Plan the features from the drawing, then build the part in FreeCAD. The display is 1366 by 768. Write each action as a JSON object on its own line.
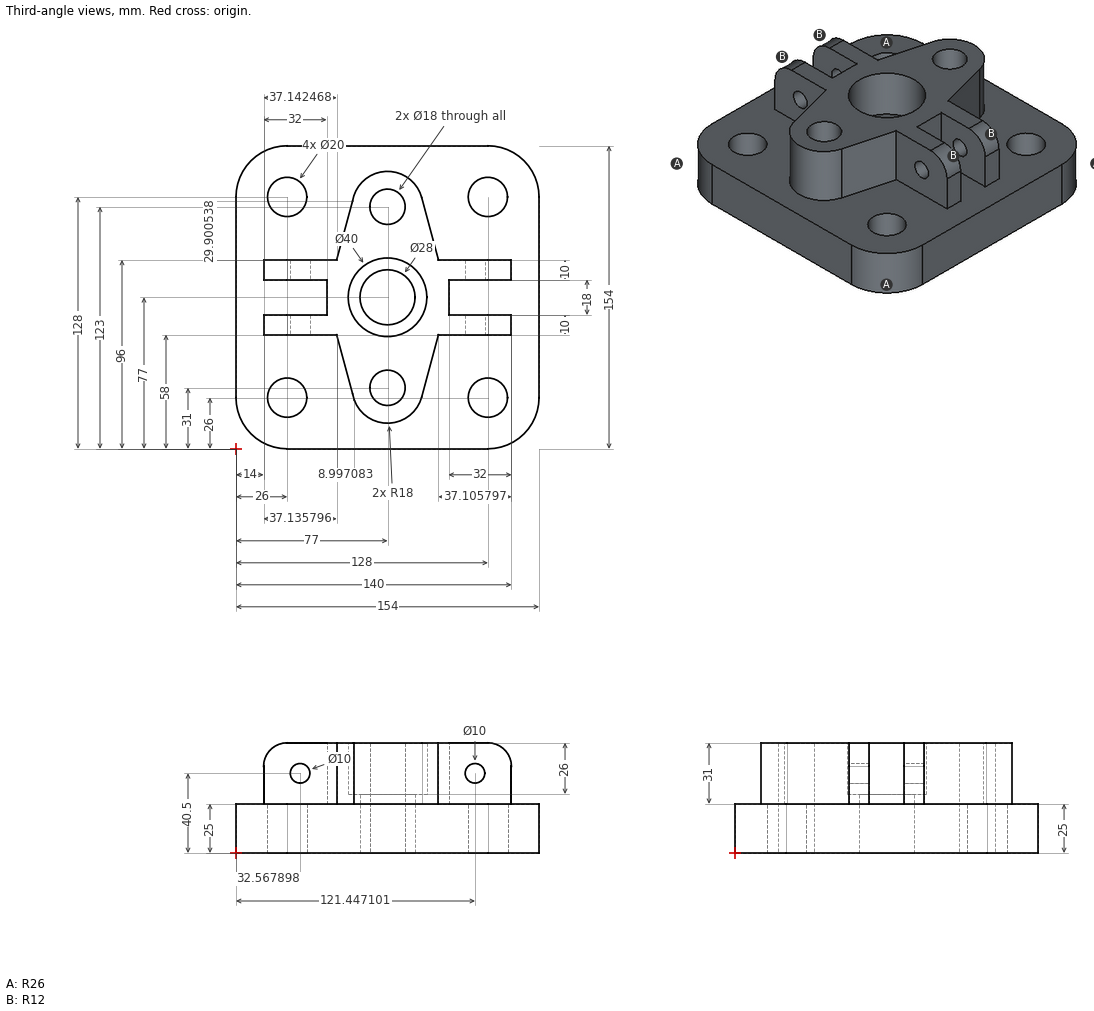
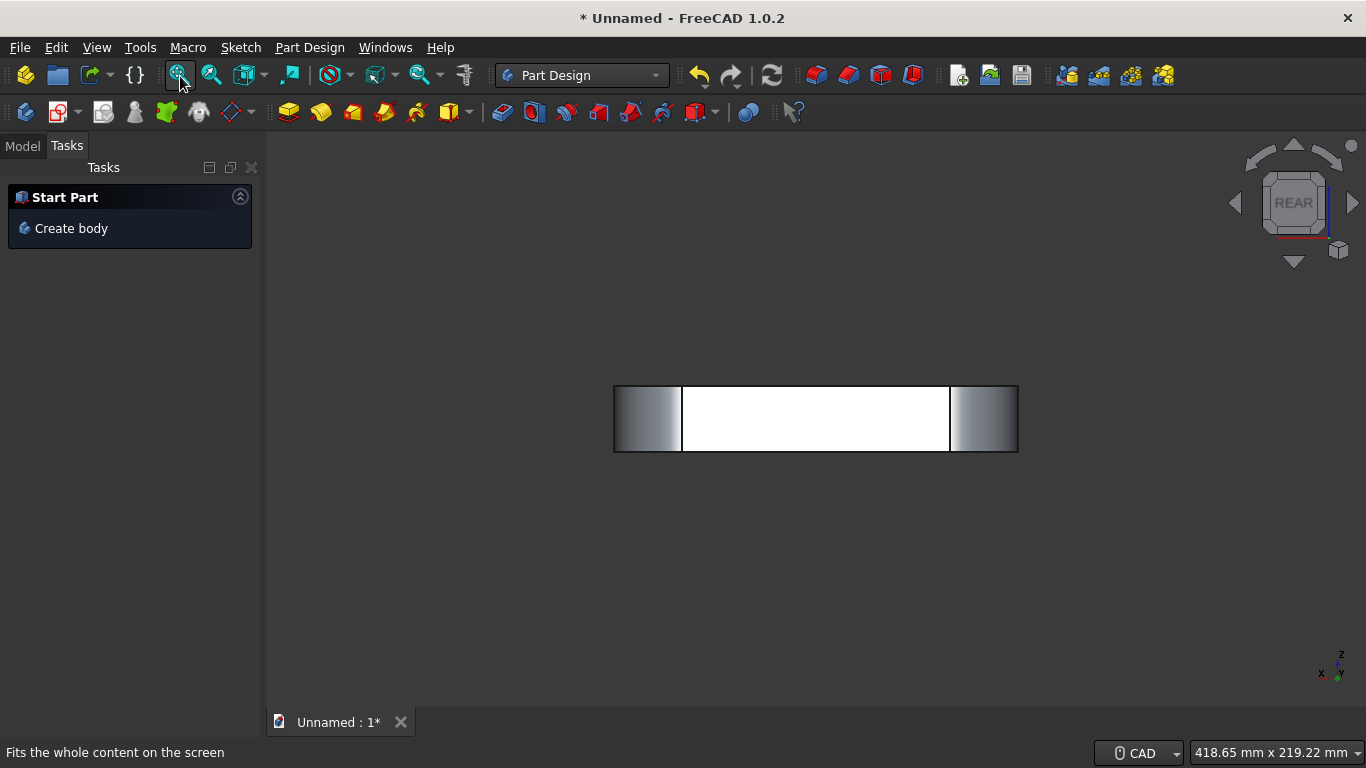
{"action": "key", "text": "0"}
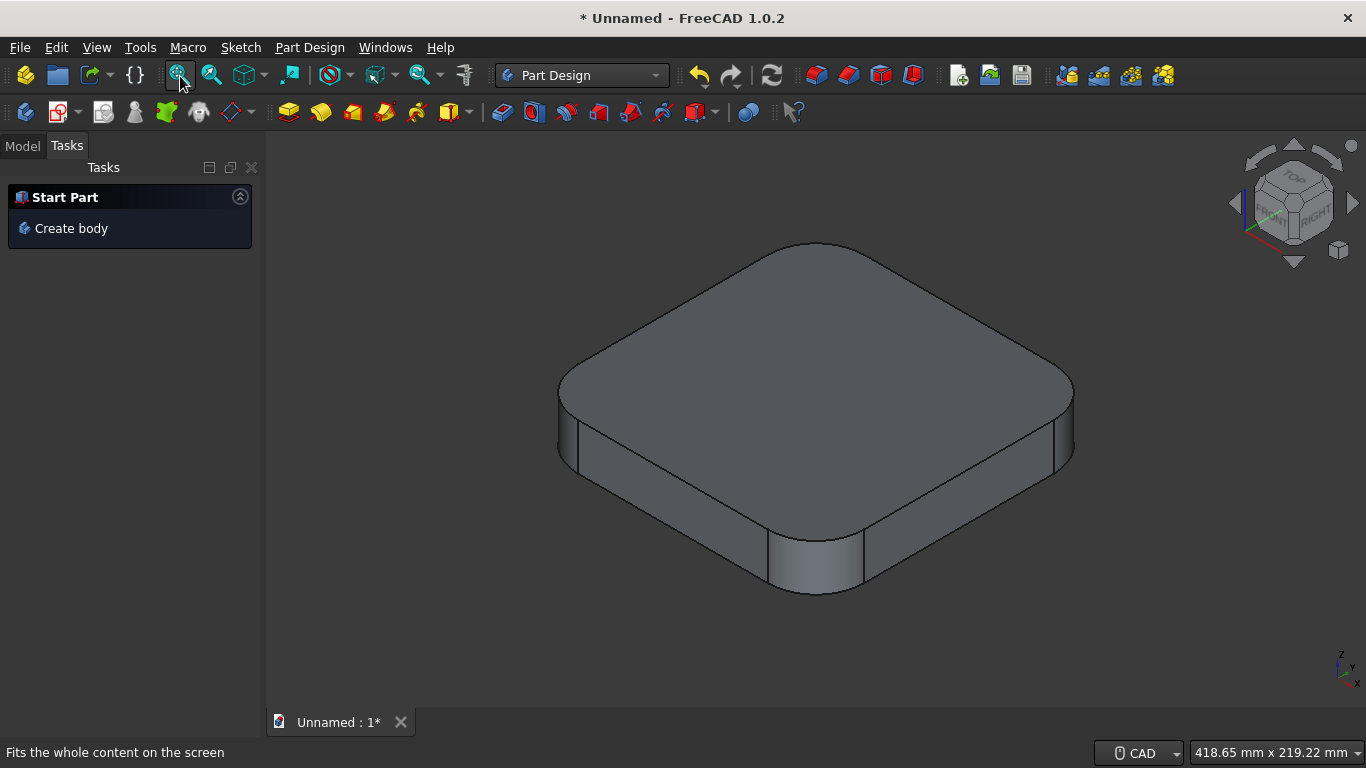
{"action": "left_click", "coordinate": [816, 391]}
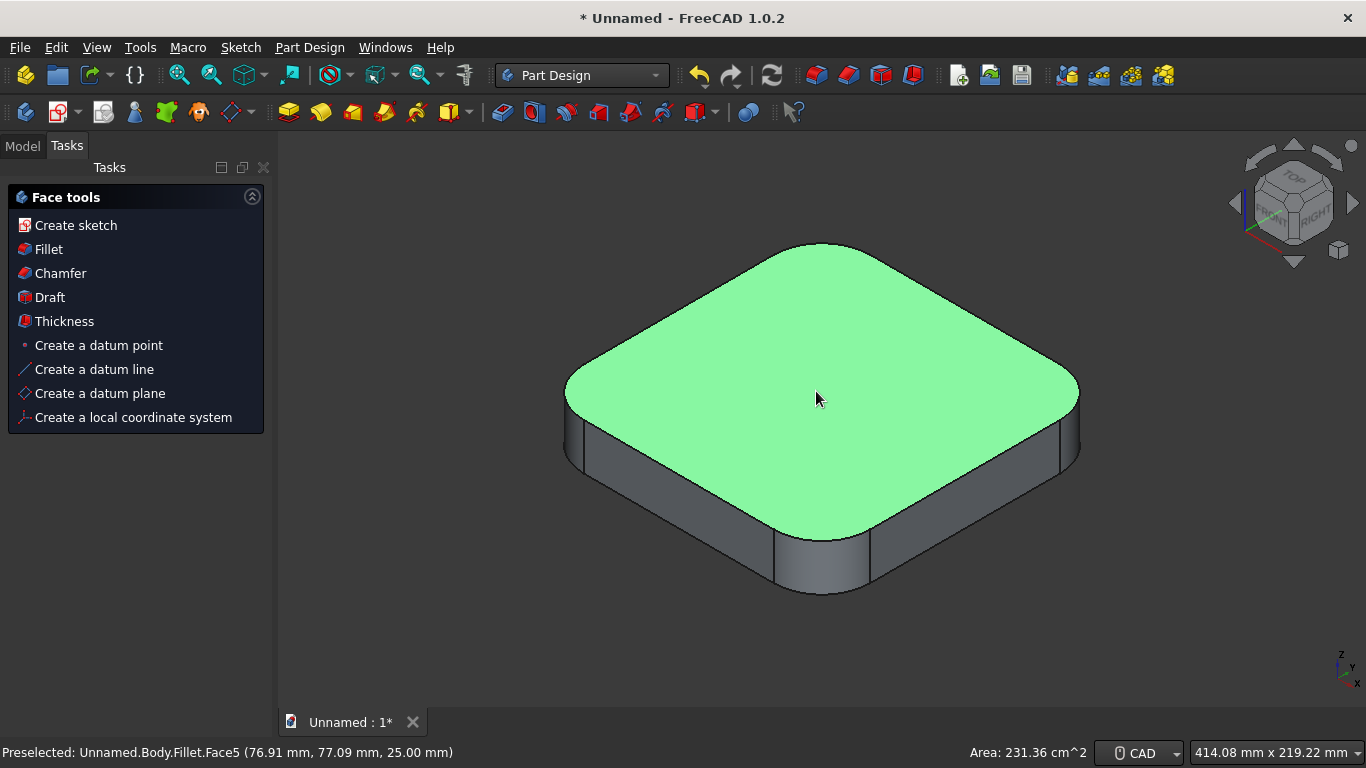
{"action": "left_click", "coordinate": [58, 112]}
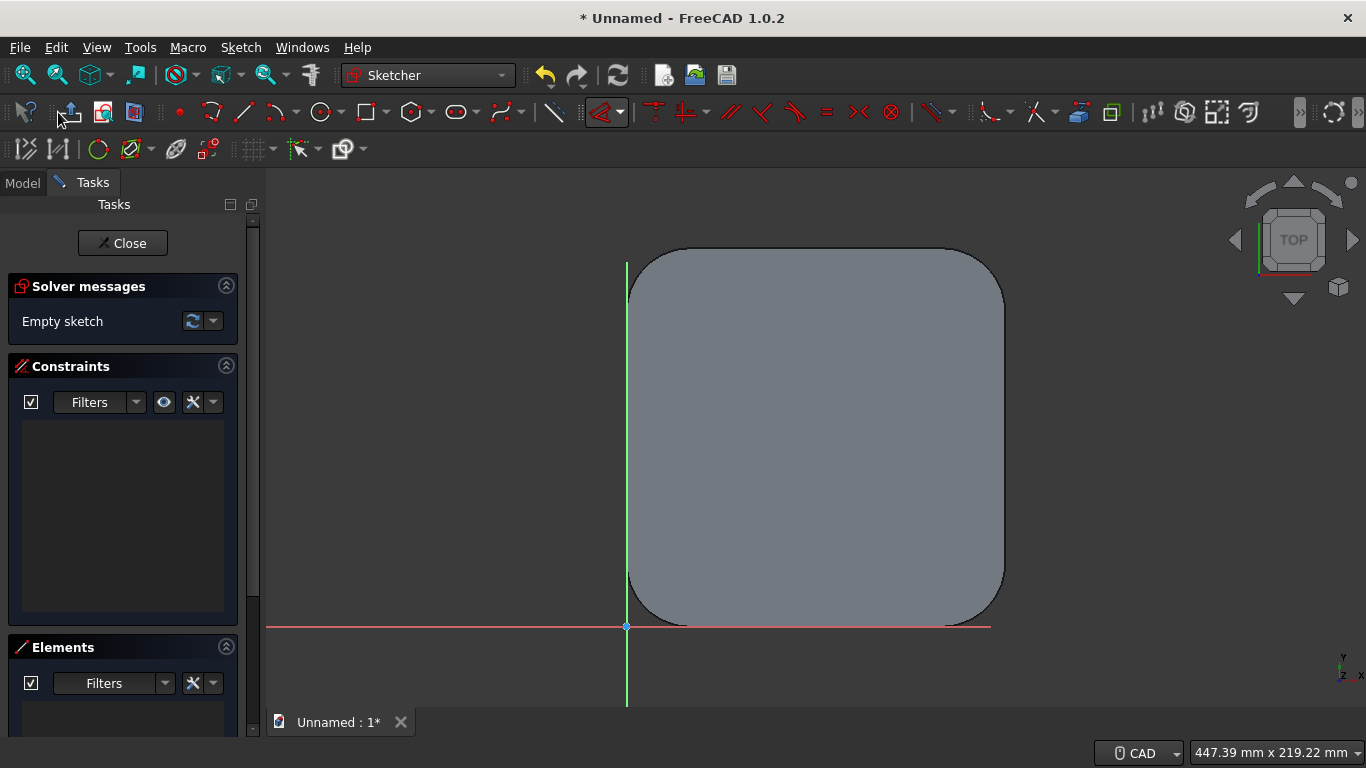
{"action": "left_click", "coordinate": [322, 112]}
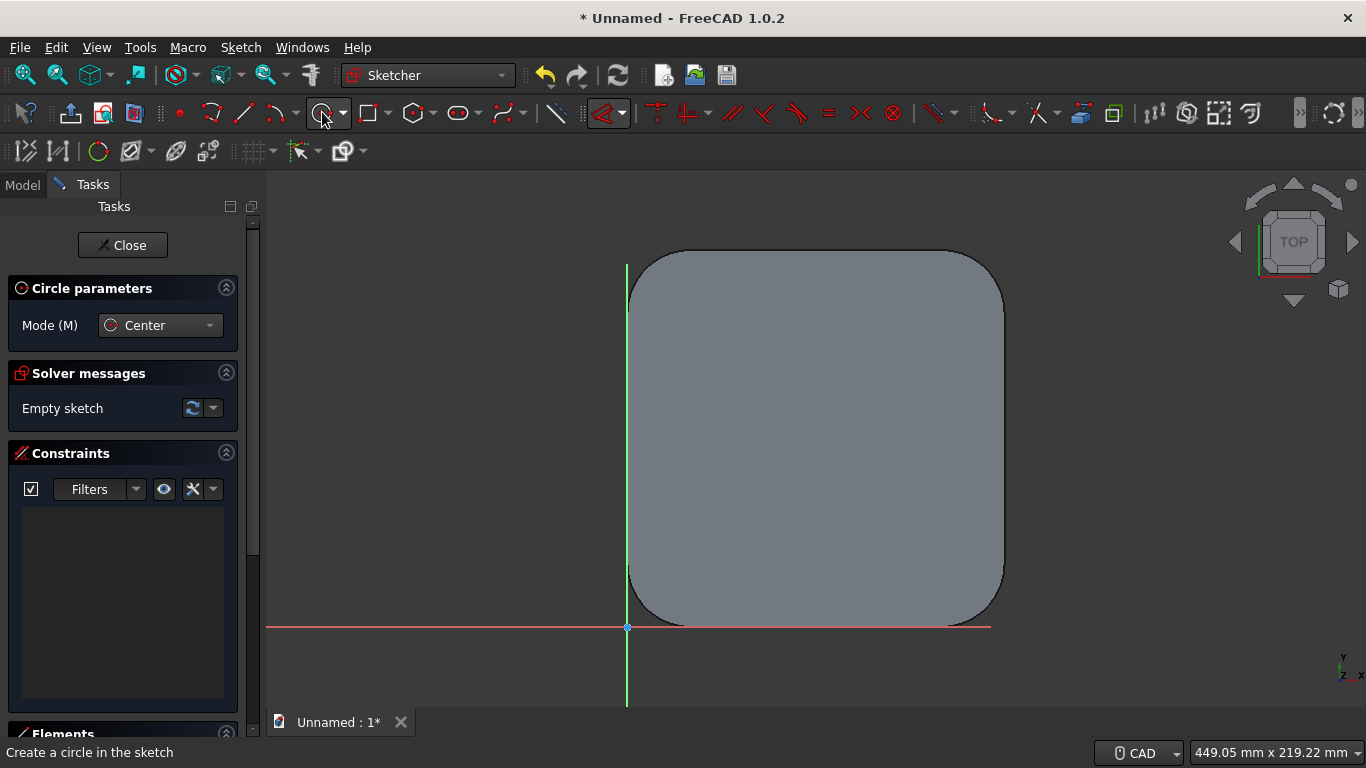
{"action": "left_click", "coordinate": [691, 314]}
{"action": "left_click", "coordinate": [708, 296]}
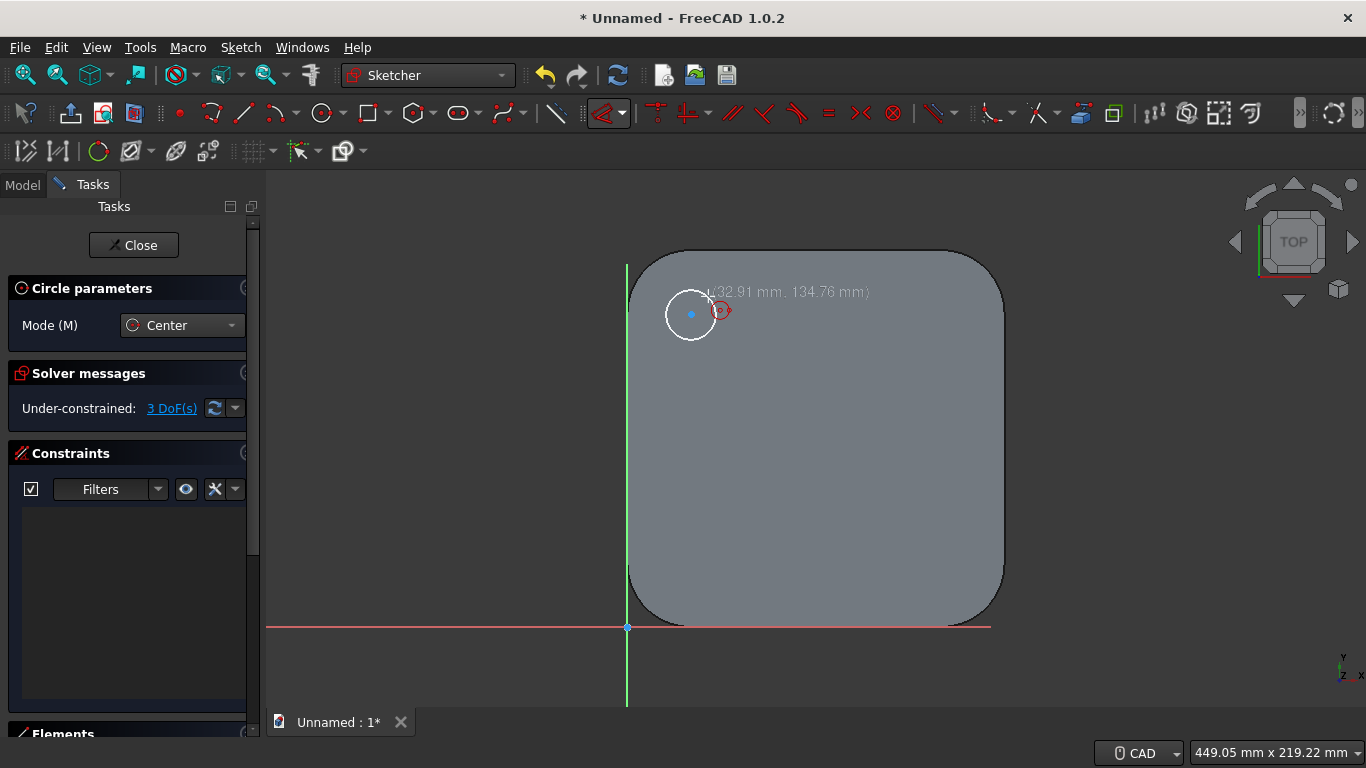
{"action": "left_click", "coordinate": [941, 314]}
{"action": "left_click", "coordinate": [958, 296]}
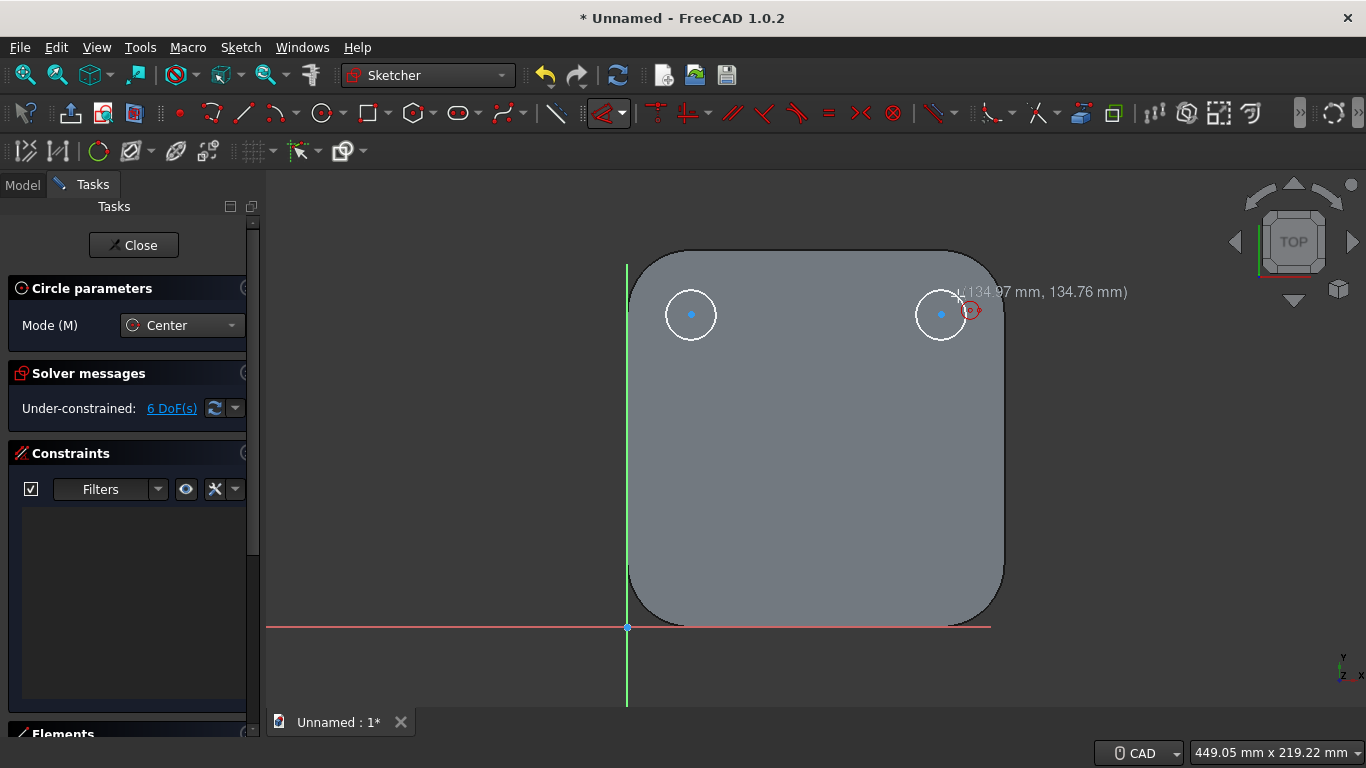
{"action": "left_click", "coordinate": [941, 563]}
{"action": "left_click", "coordinate": [958, 546]}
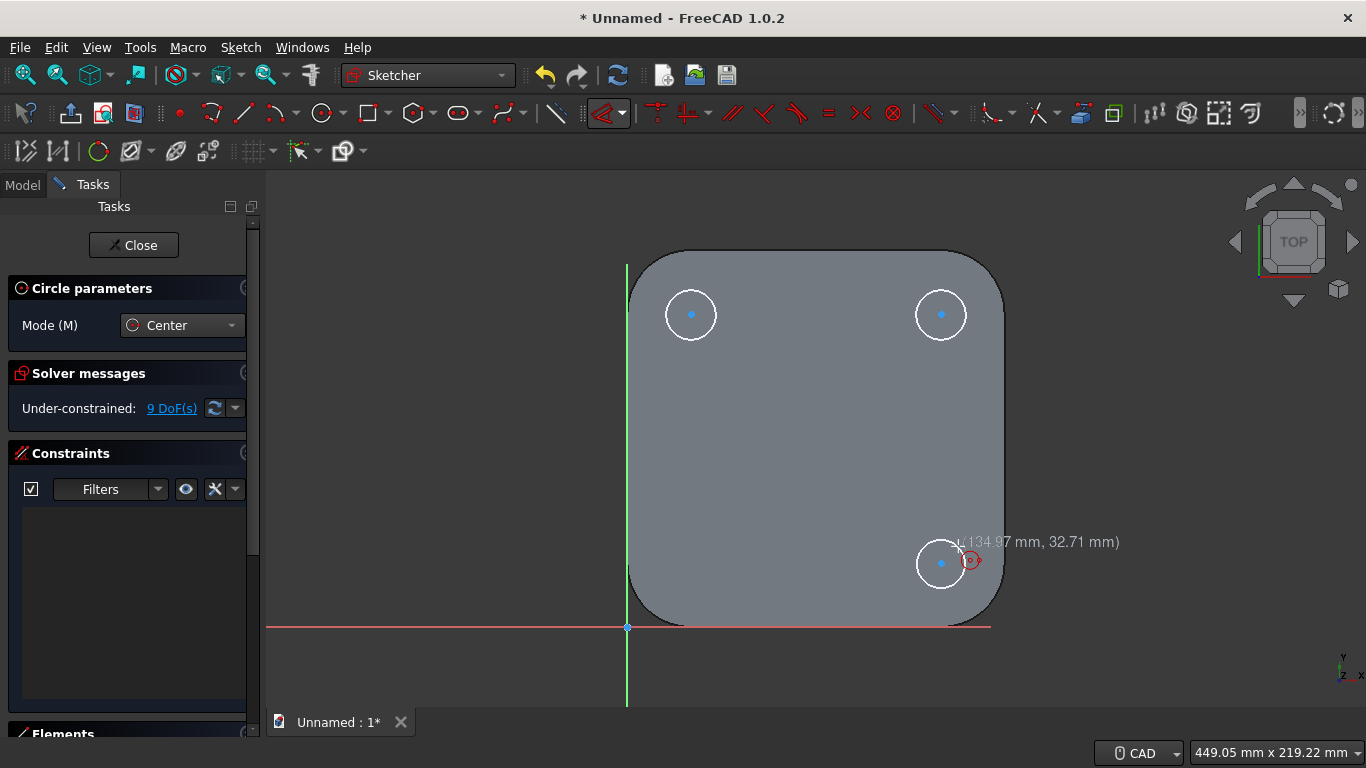
{"action": "left_click", "coordinate": [691, 563]}
{"action": "left_click", "coordinate": [708, 546]}
{"action": "key", "text": "Escape"}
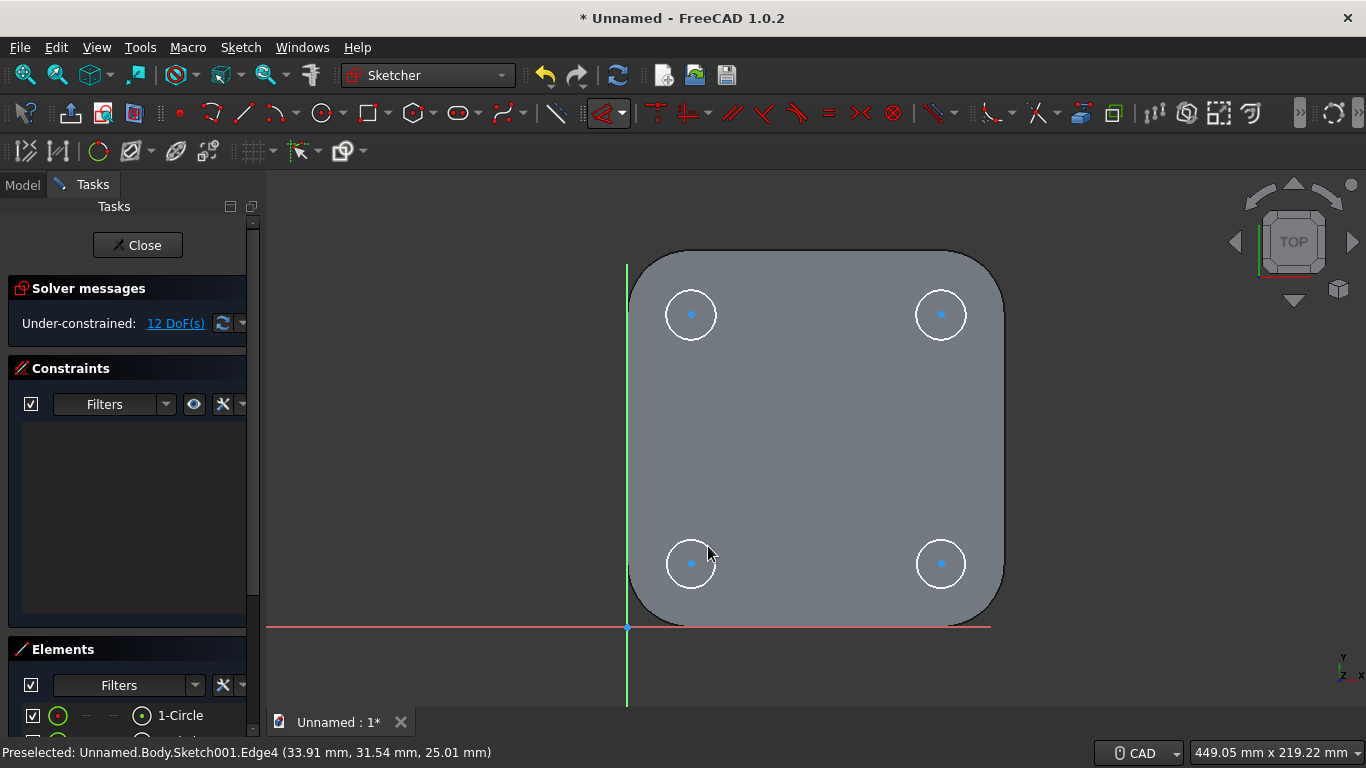
{"action": "left_click", "coordinate": [708, 297]}